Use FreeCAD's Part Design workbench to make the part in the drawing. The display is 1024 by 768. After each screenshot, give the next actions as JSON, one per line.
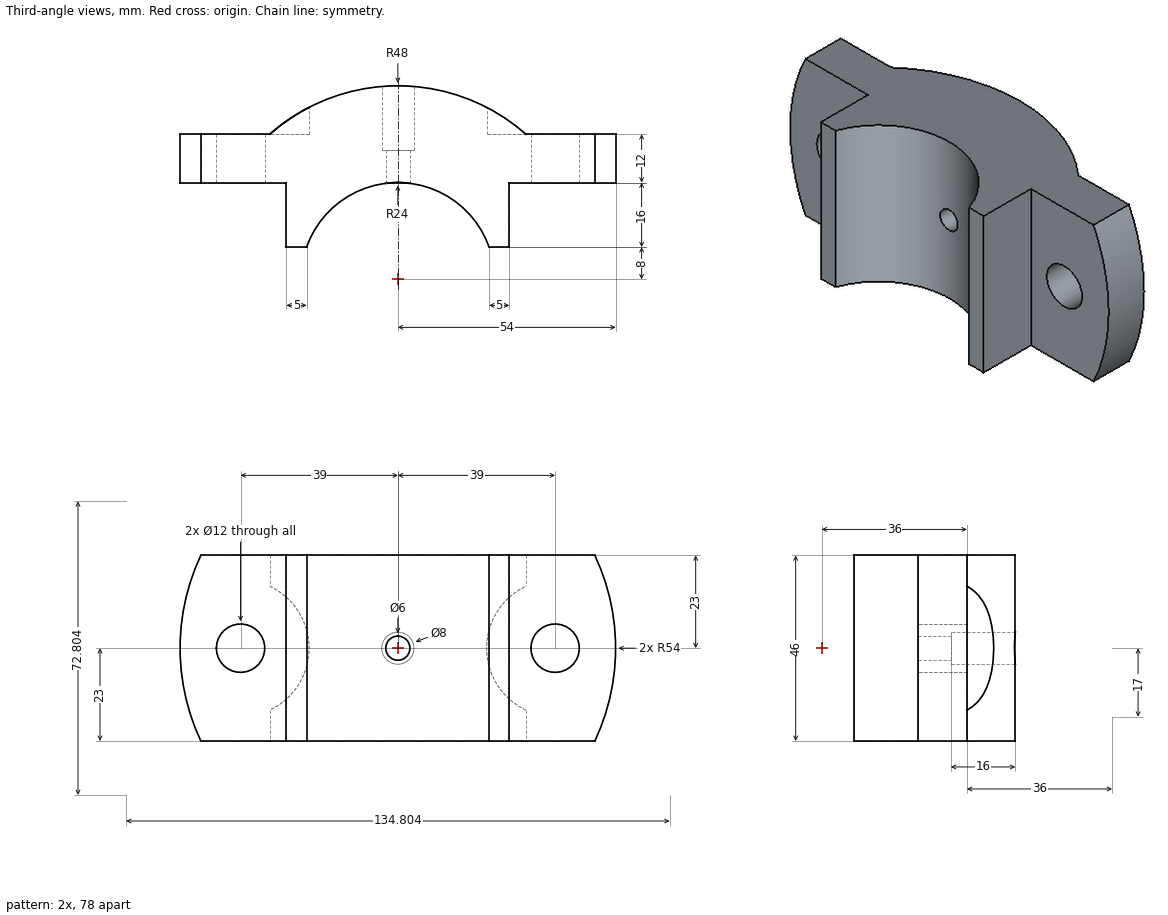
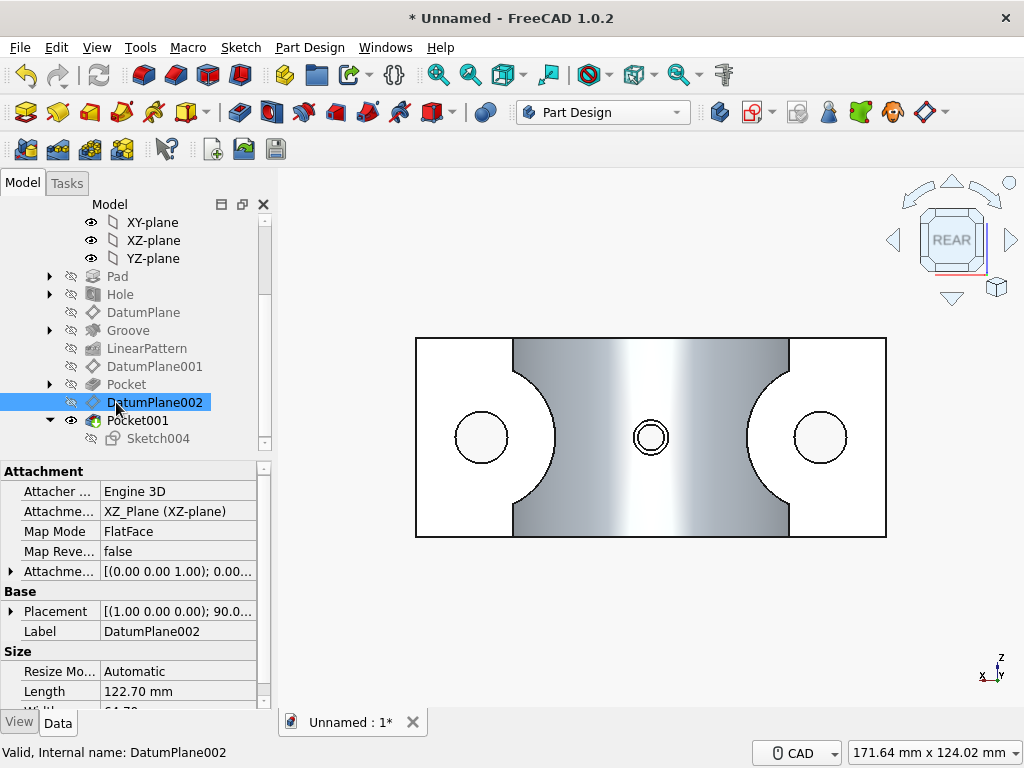
{"action": "left_click", "coordinate": [836, 379]}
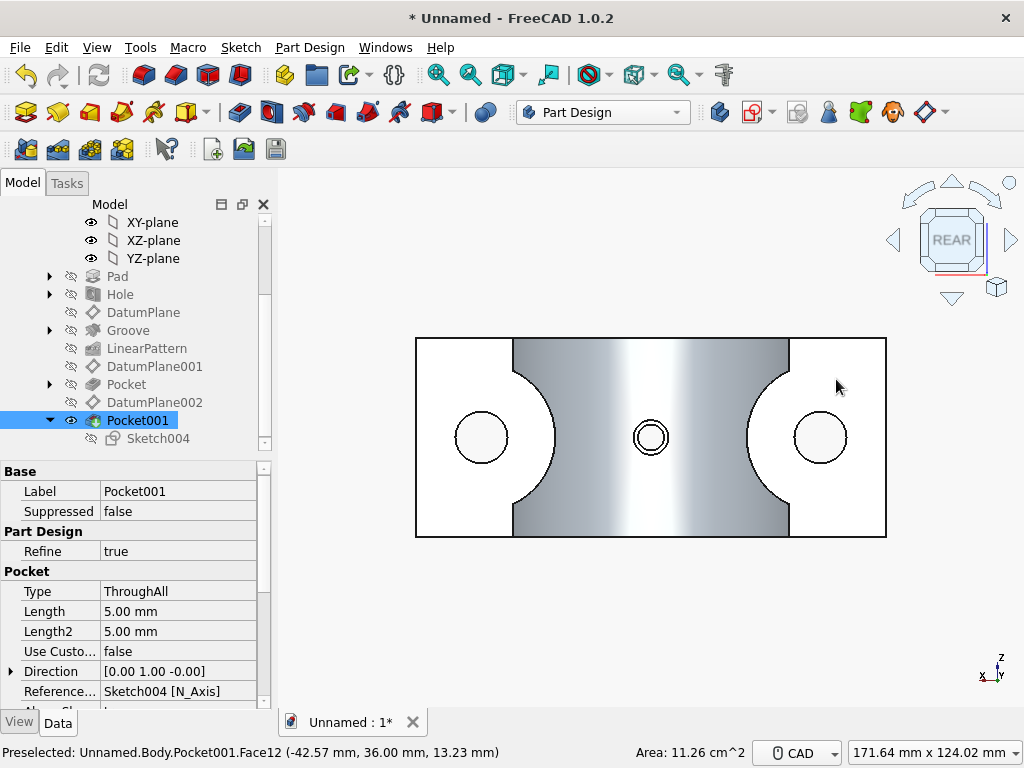
{"action": "left_click", "coordinate": [752, 112]}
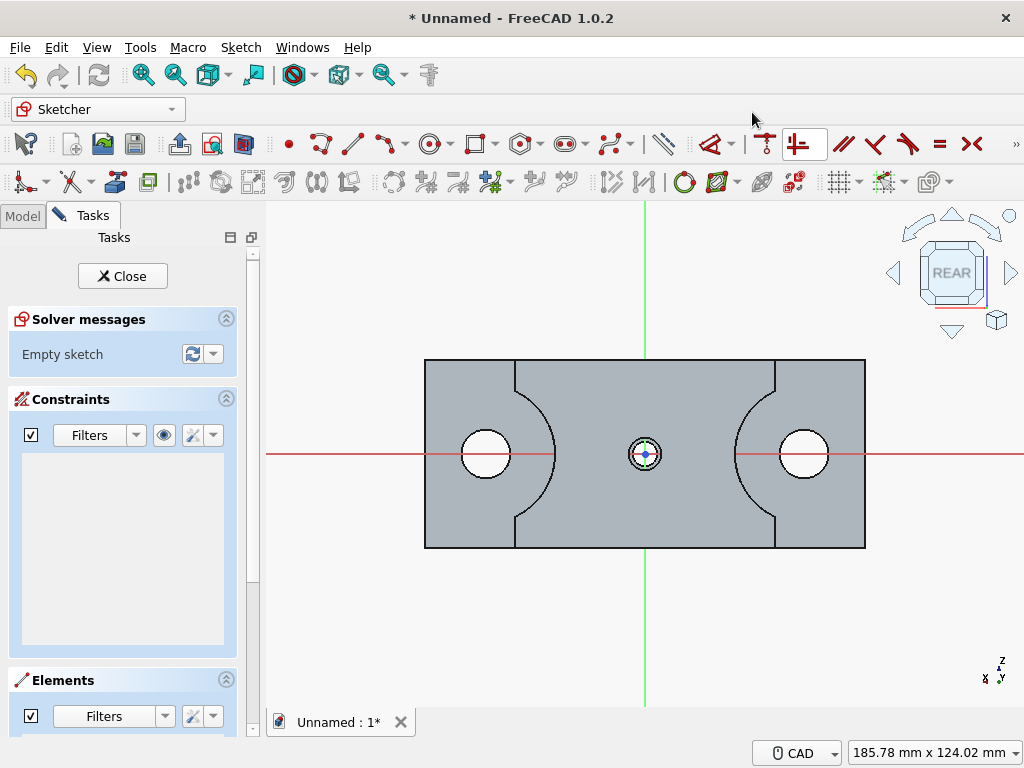
{"action": "scroll", "coordinate": [437, 454], "scroll_direction": "down", "scroll_amount": 2}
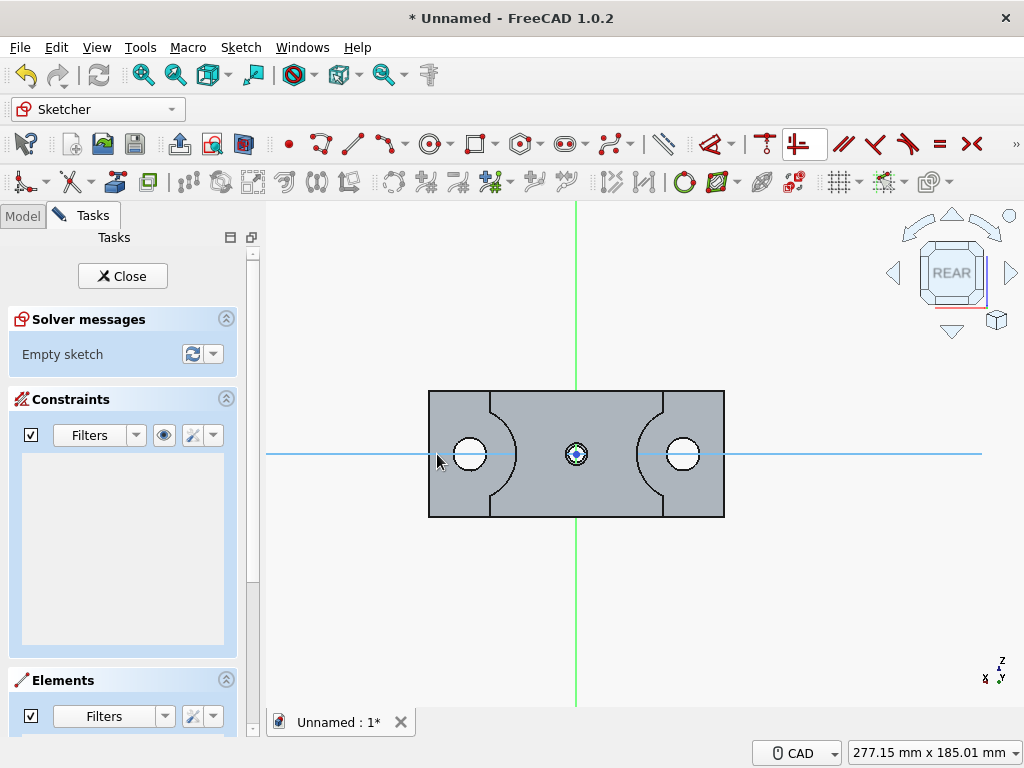
{"action": "left_click", "coordinate": [498, 144]}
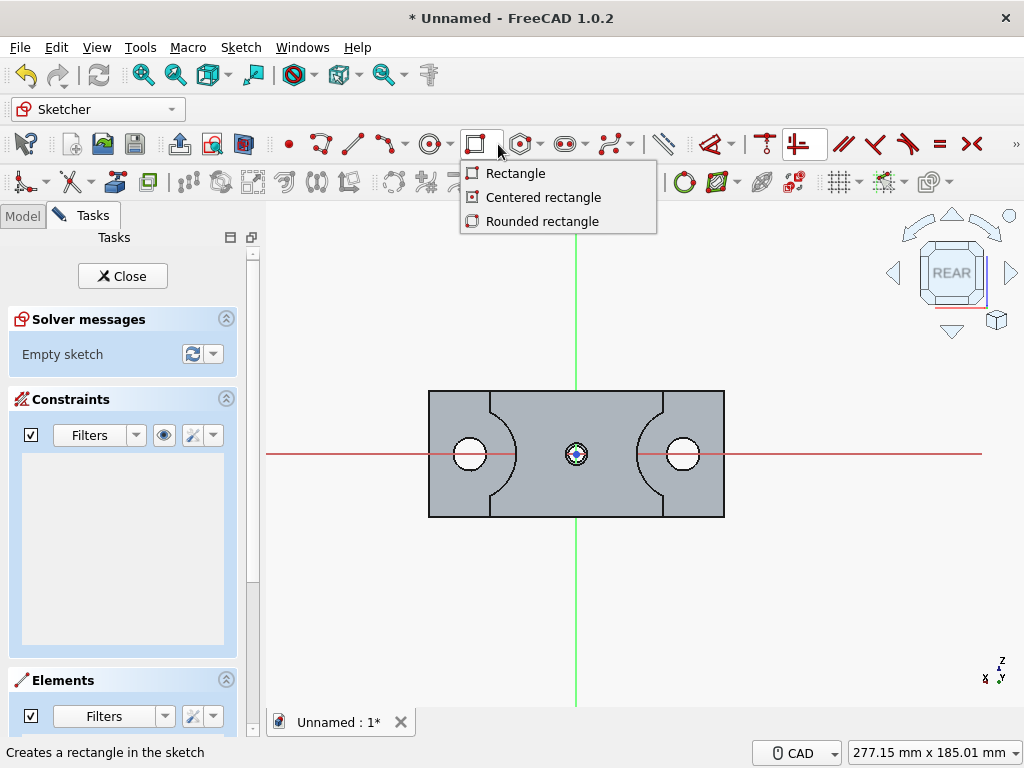
{"action": "left_click", "coordinate": [558, 197]}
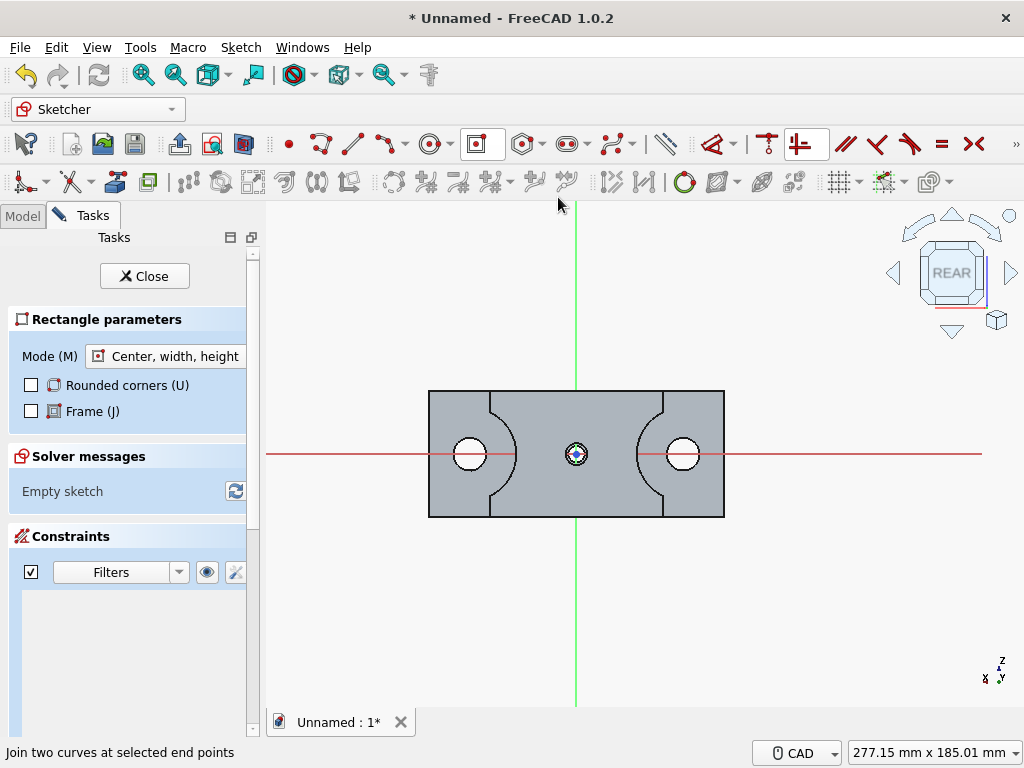
{"action": "left_click", "coordinate": [577, 454]}
{"action": "mouse_move", "coordinate": [761, 355]}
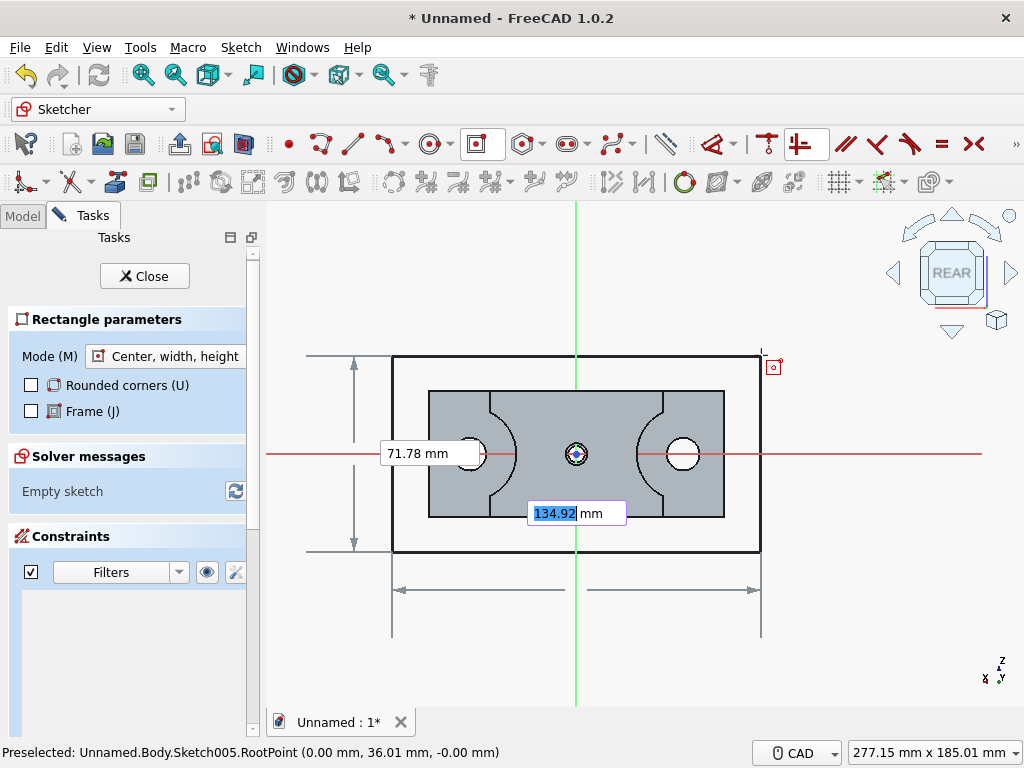
{"action": "type", "text": "134.804"}
{"action": "key", "text": "Tab"}
{"action": "type", "text": "72.804"}
{"action": "key", "text": "Return"}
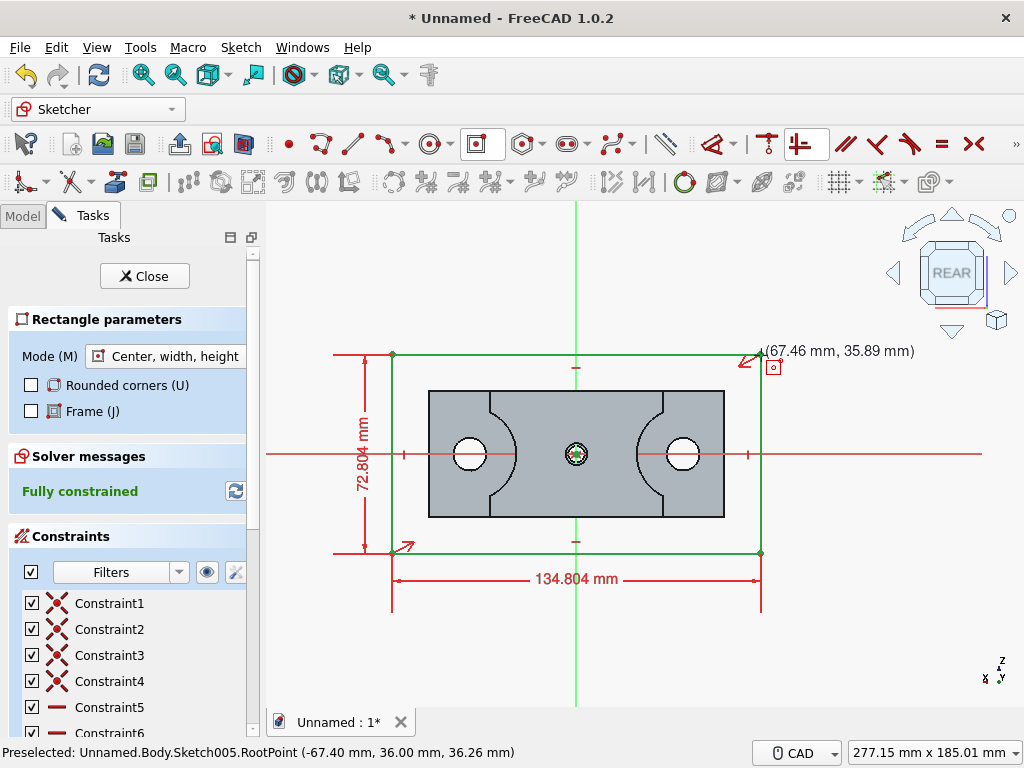
{"action": "left_click", "coordinate": [354, 144]}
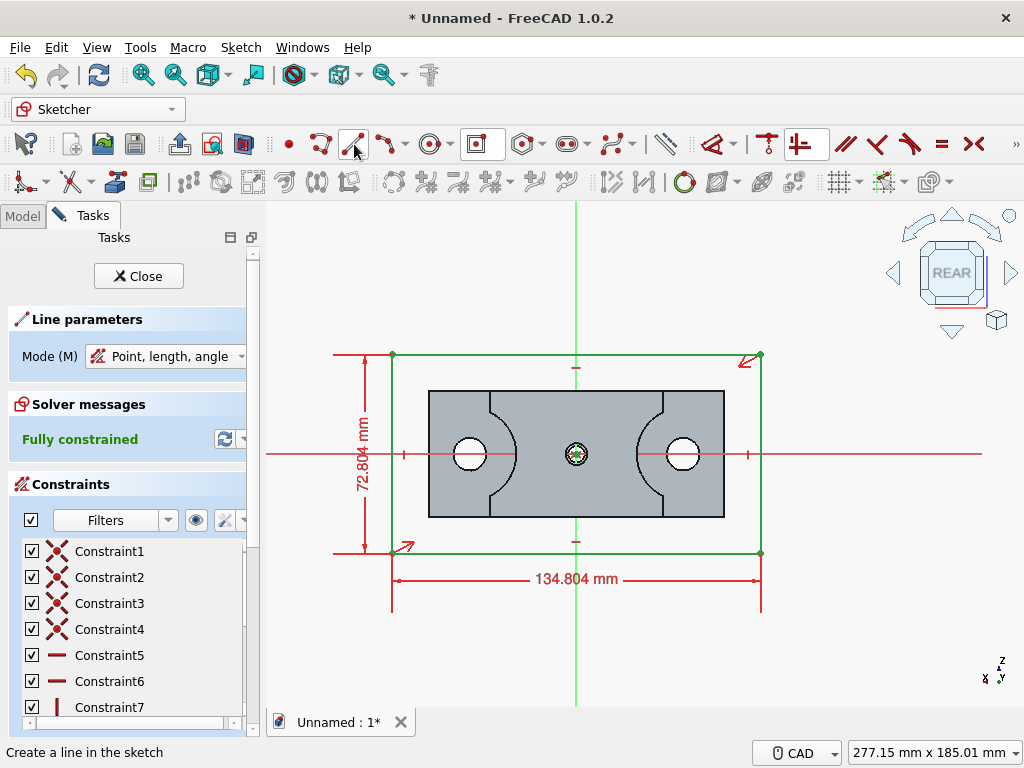
{"action": "left_click", "coordinate": [710, 517]}
{"action": "left_click", "coordinate": [443, 517]}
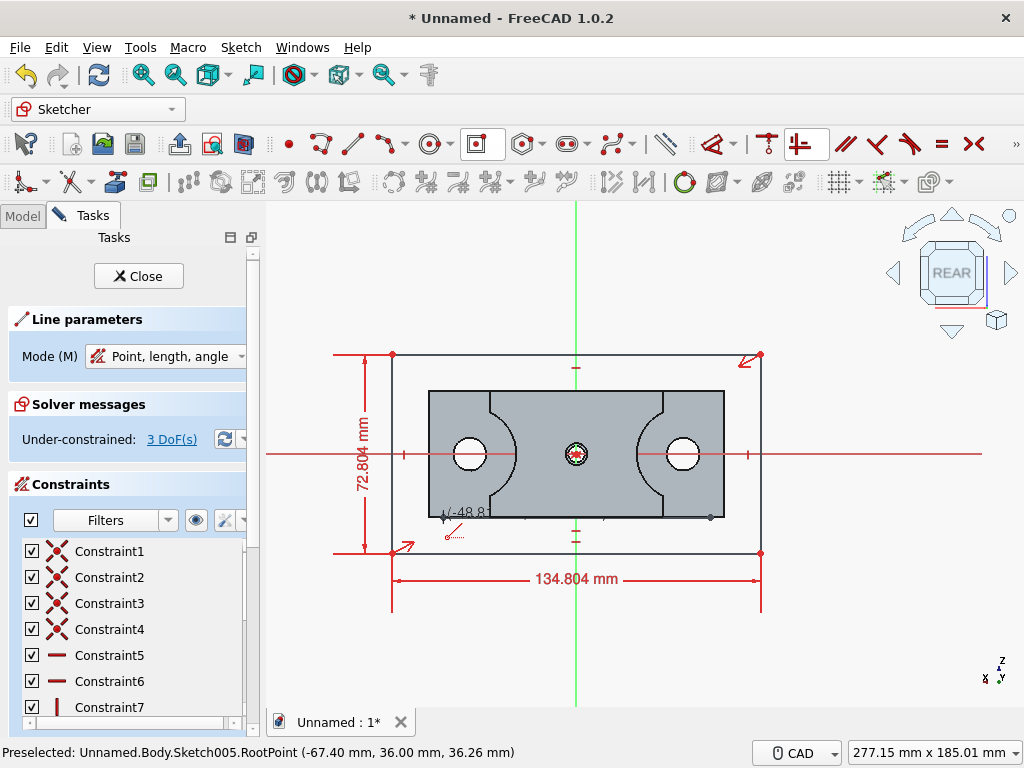
{"action": "left_click", "coordinate": [443, 391]}
{"action": "left_click", "coordinate": [710, 391]}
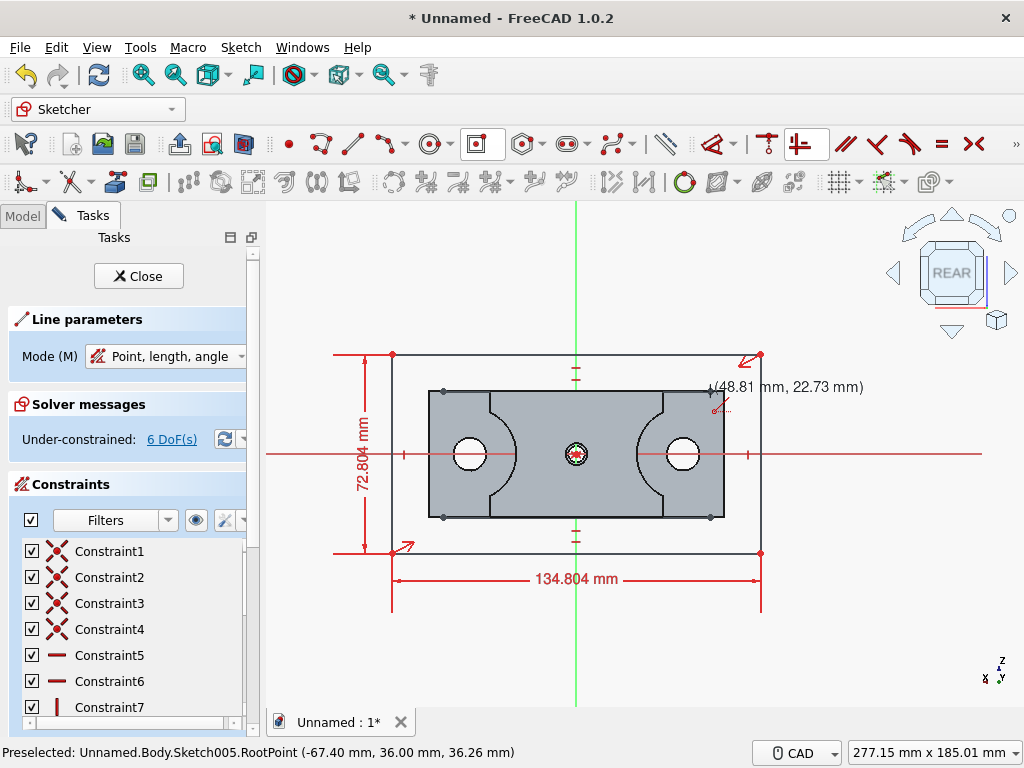
{"action": "left_click", "coordinate": [386, 144]}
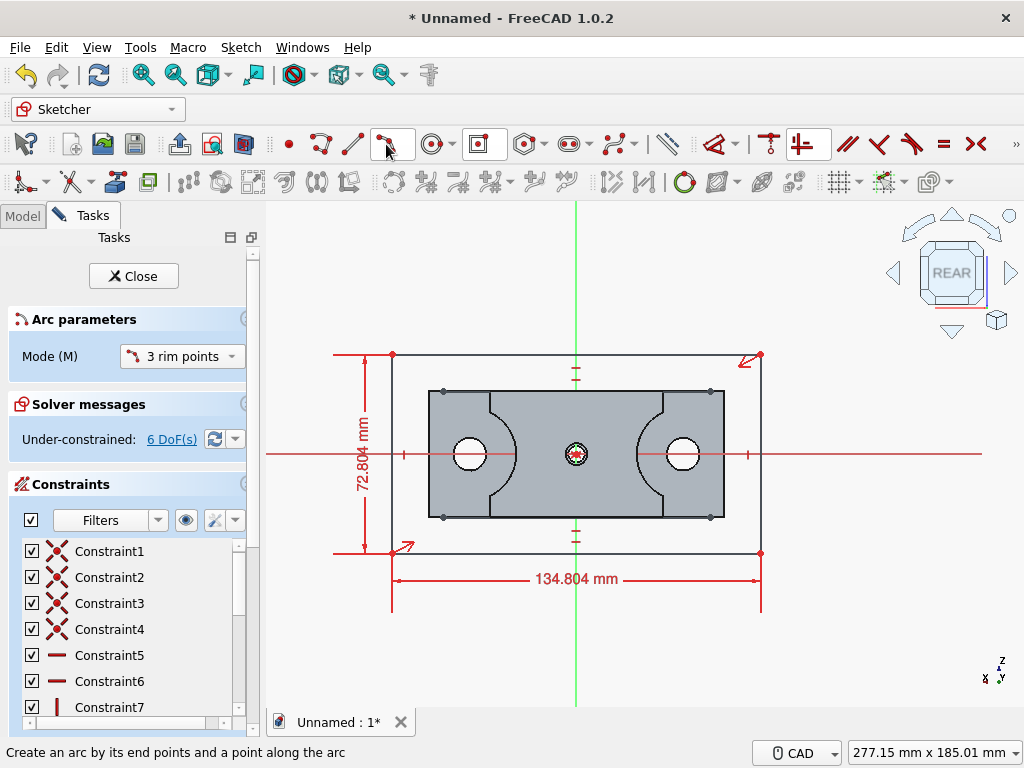
{"action": "left_click", "coordinate": [443, 518]}
{"action": "left_click", "coordinate": [443, 392]}